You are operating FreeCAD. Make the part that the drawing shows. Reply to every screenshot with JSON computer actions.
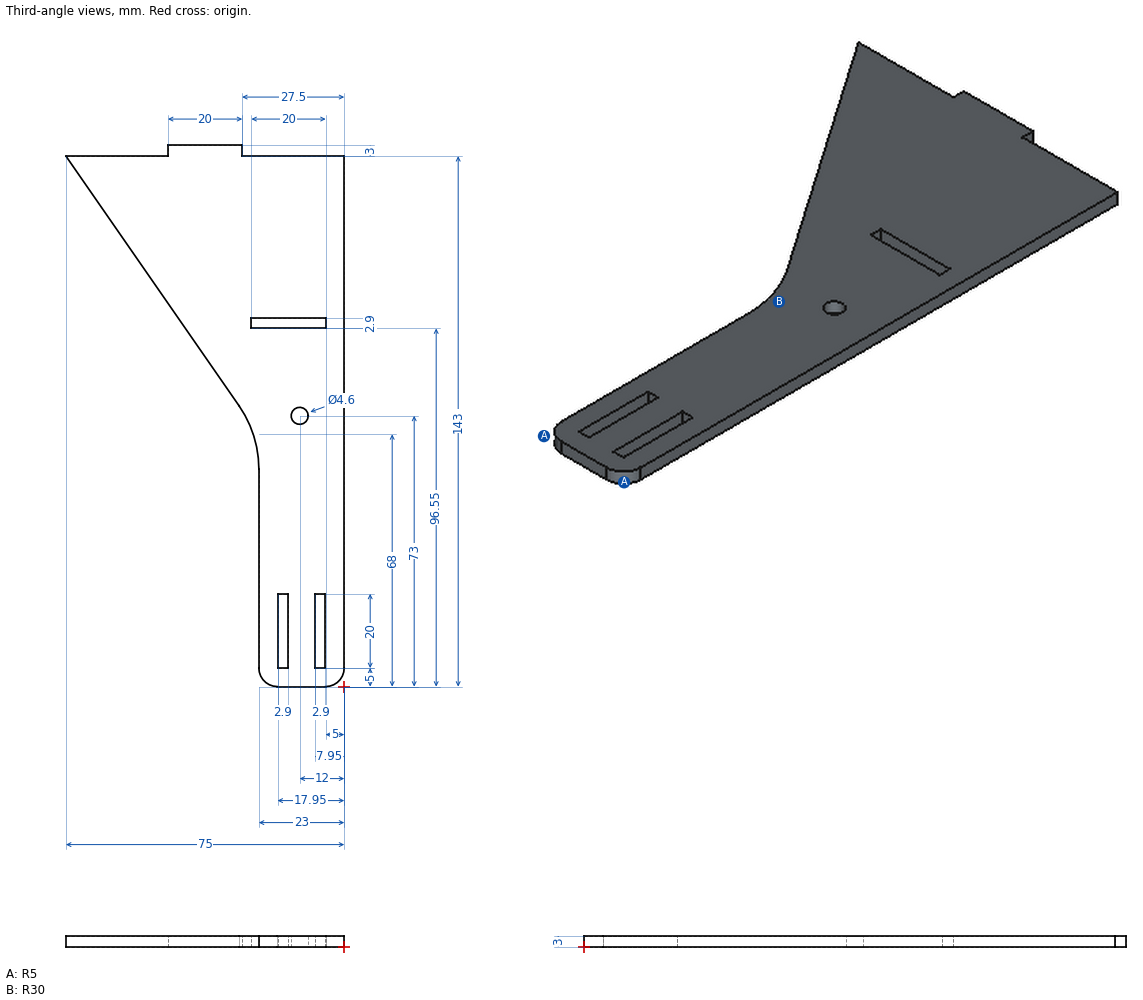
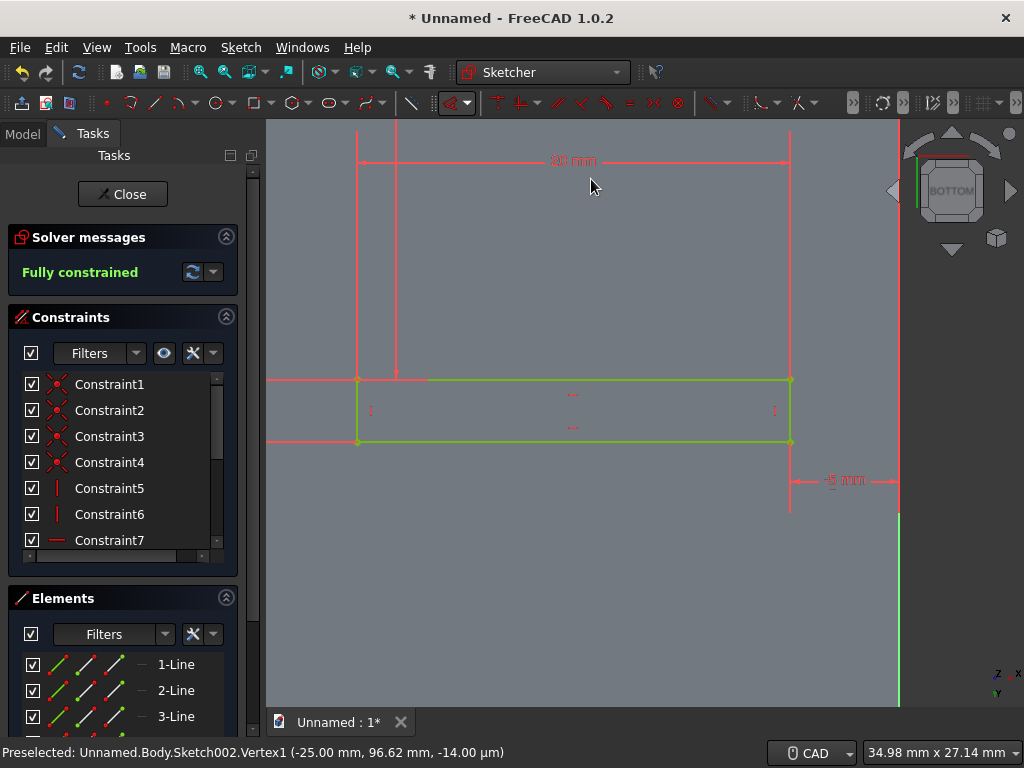
{"action": "left_click", "coordinate": [123, 194]}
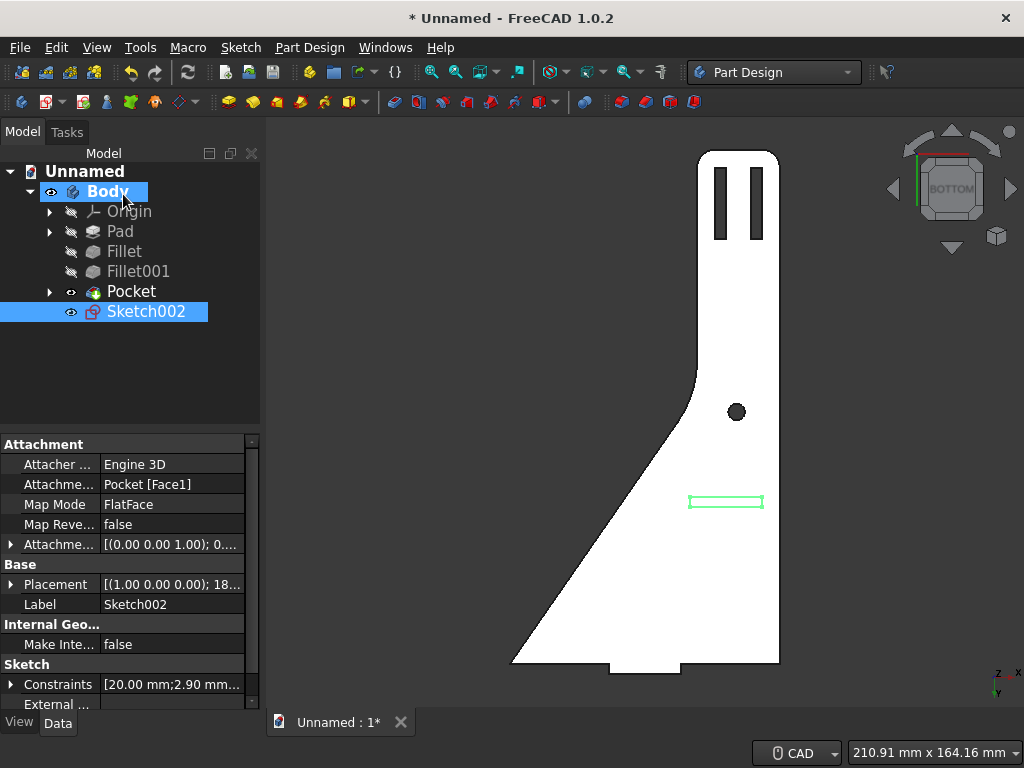
{"action": "left_click", "coordinate": [396, 102]}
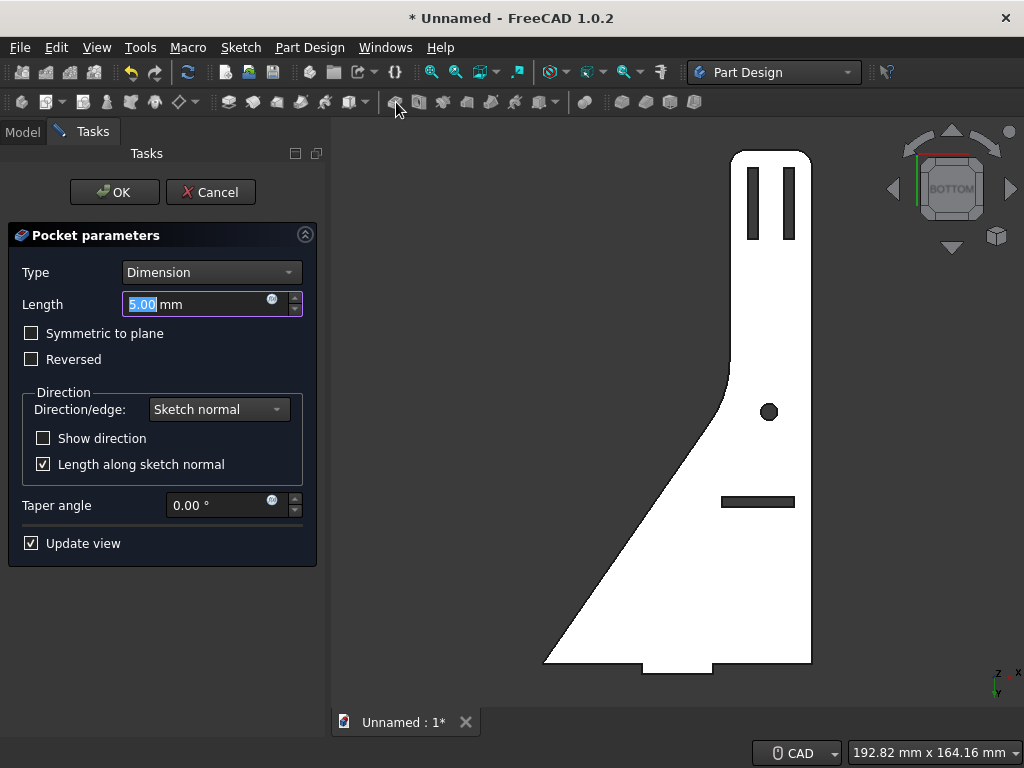
{"action": "left_click", "coordinate": [212, 272]}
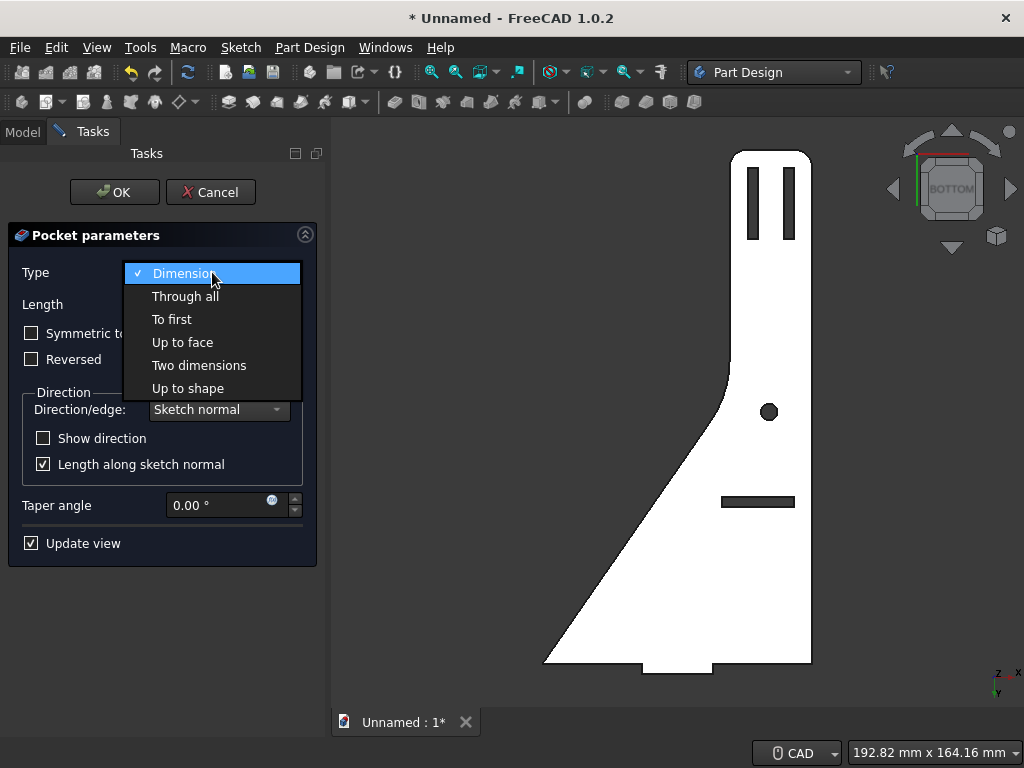
{"action": "left_click", "coordinate": [212, 296]}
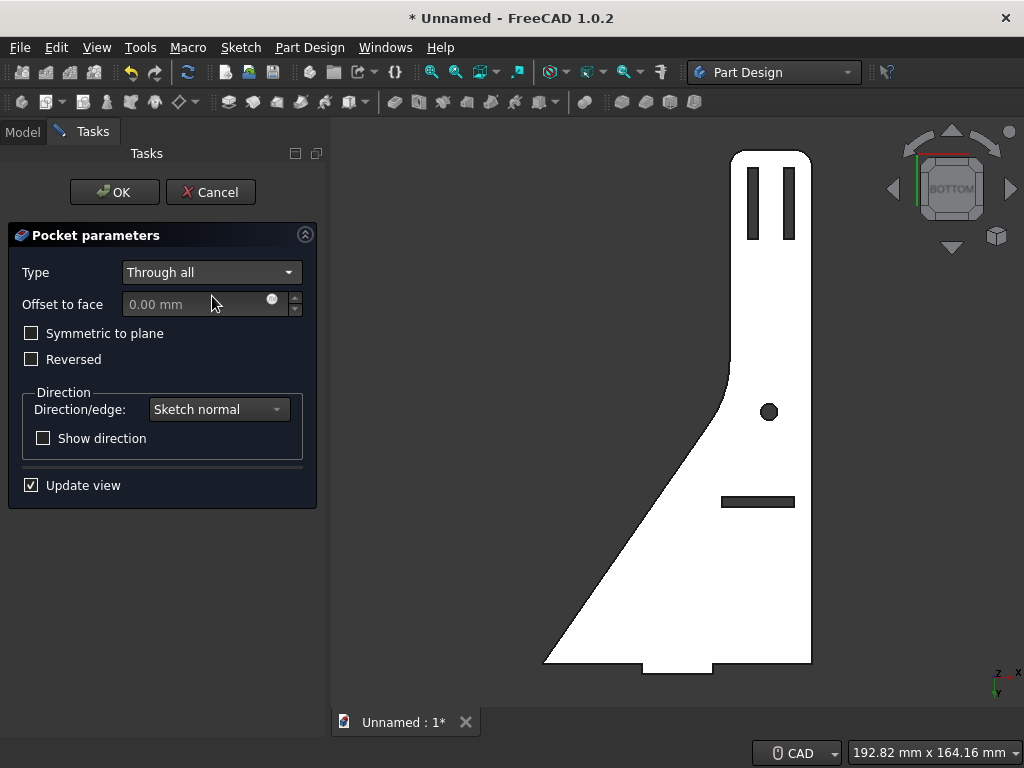
{"action": "left_click", "coordinate": [115, 192]}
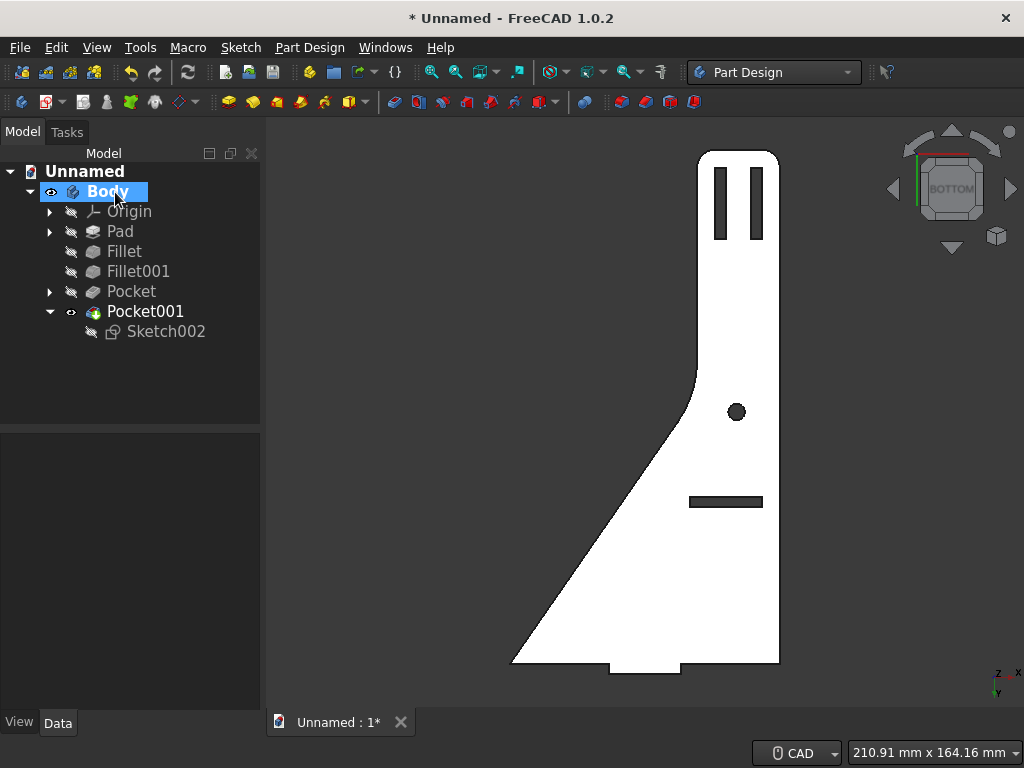
{"action": "key", "text": "0"}